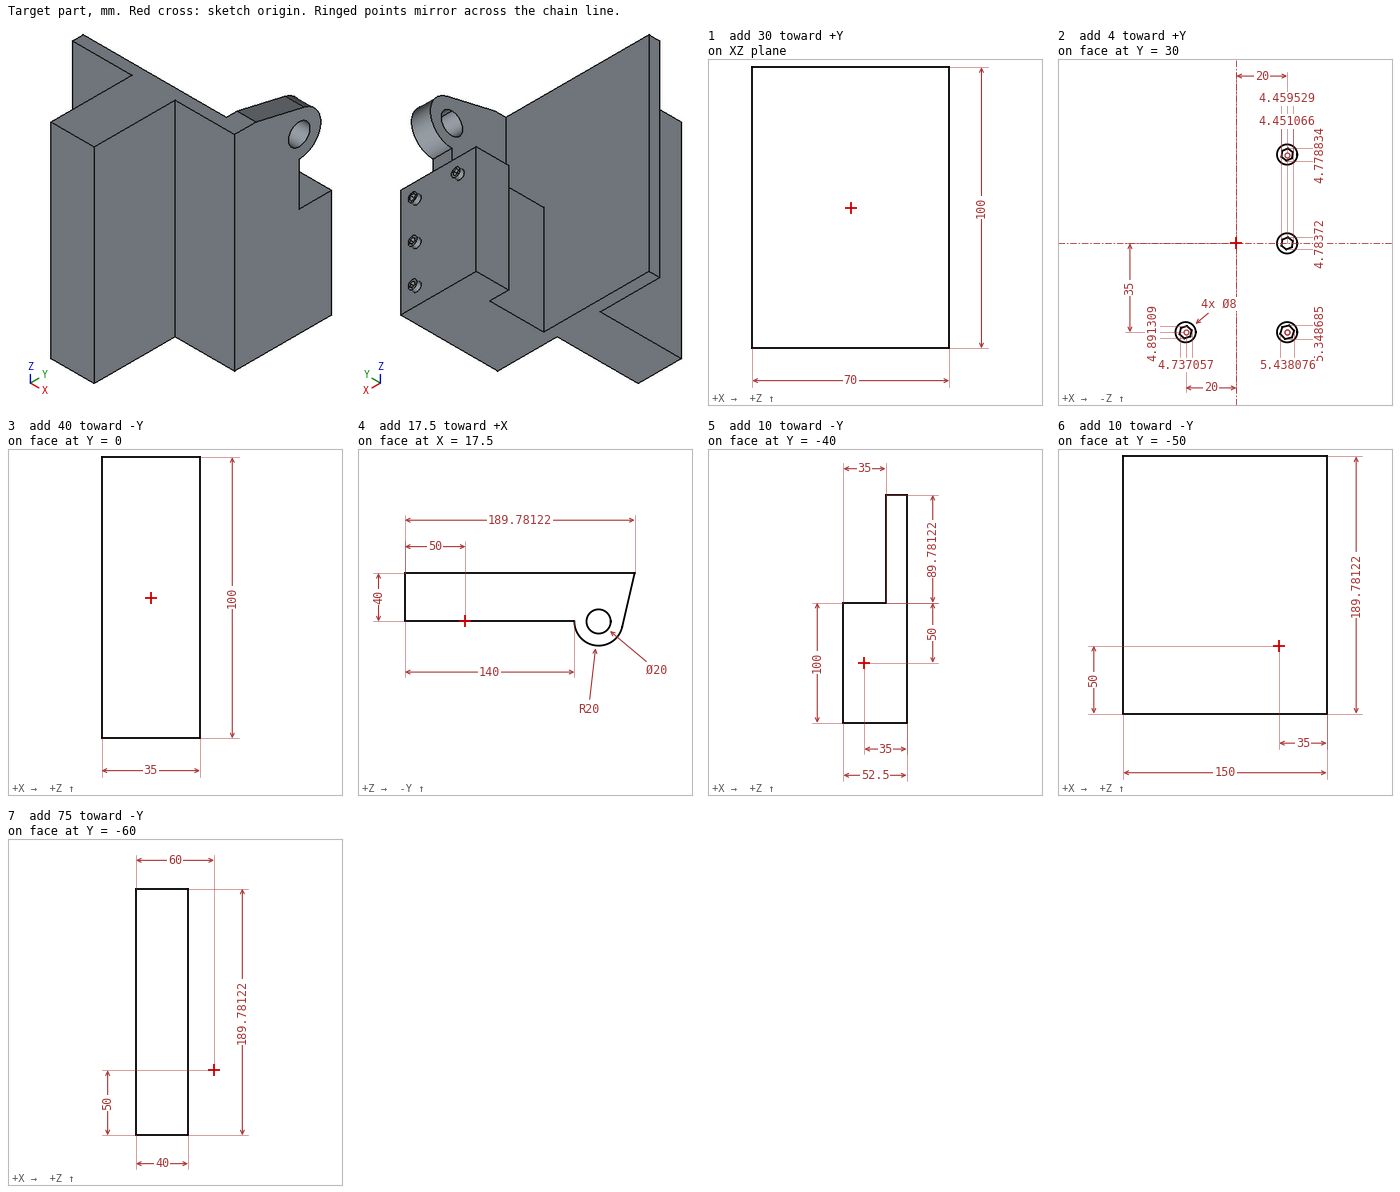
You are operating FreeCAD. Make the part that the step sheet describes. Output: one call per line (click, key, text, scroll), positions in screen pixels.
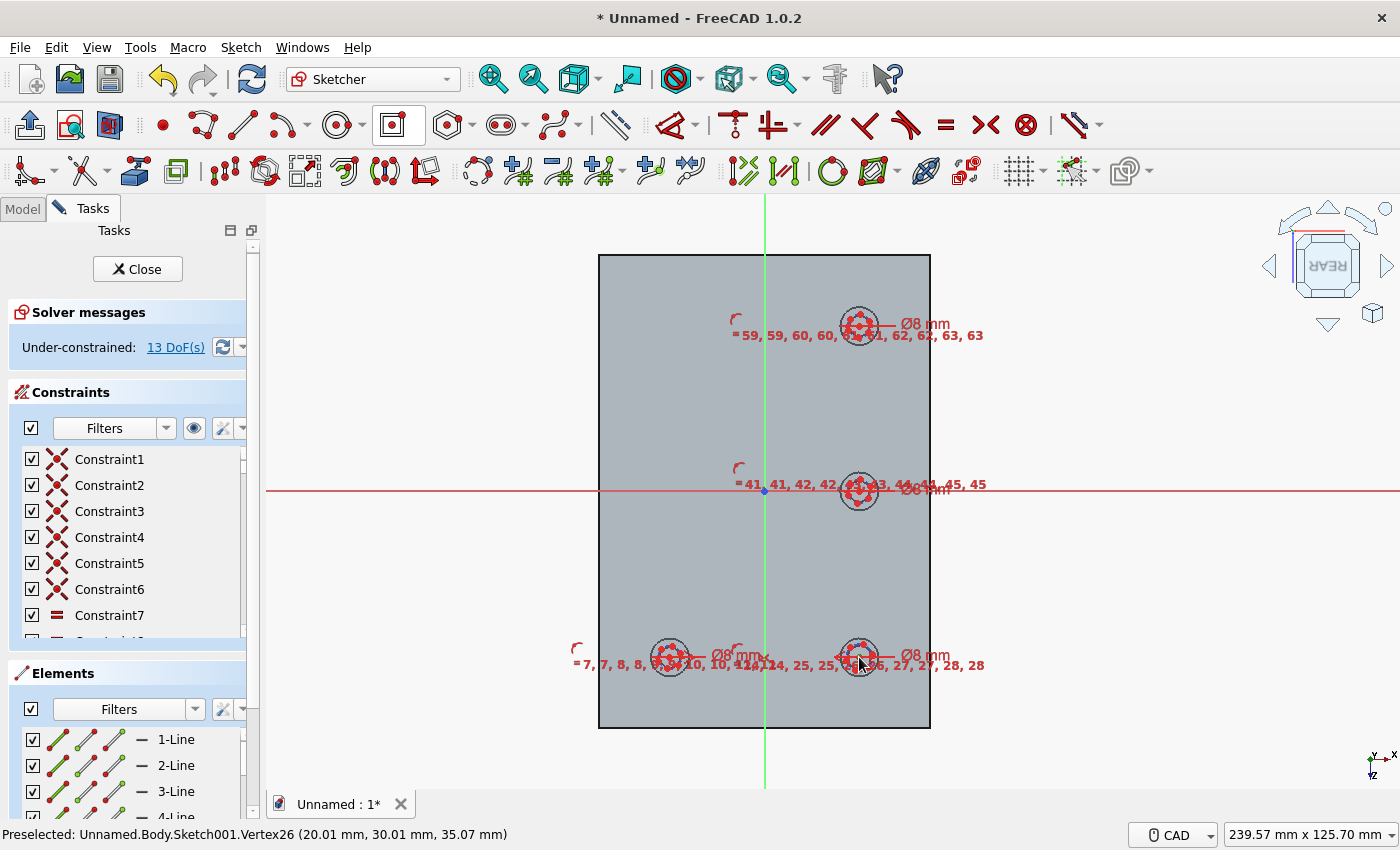
click(859, 326)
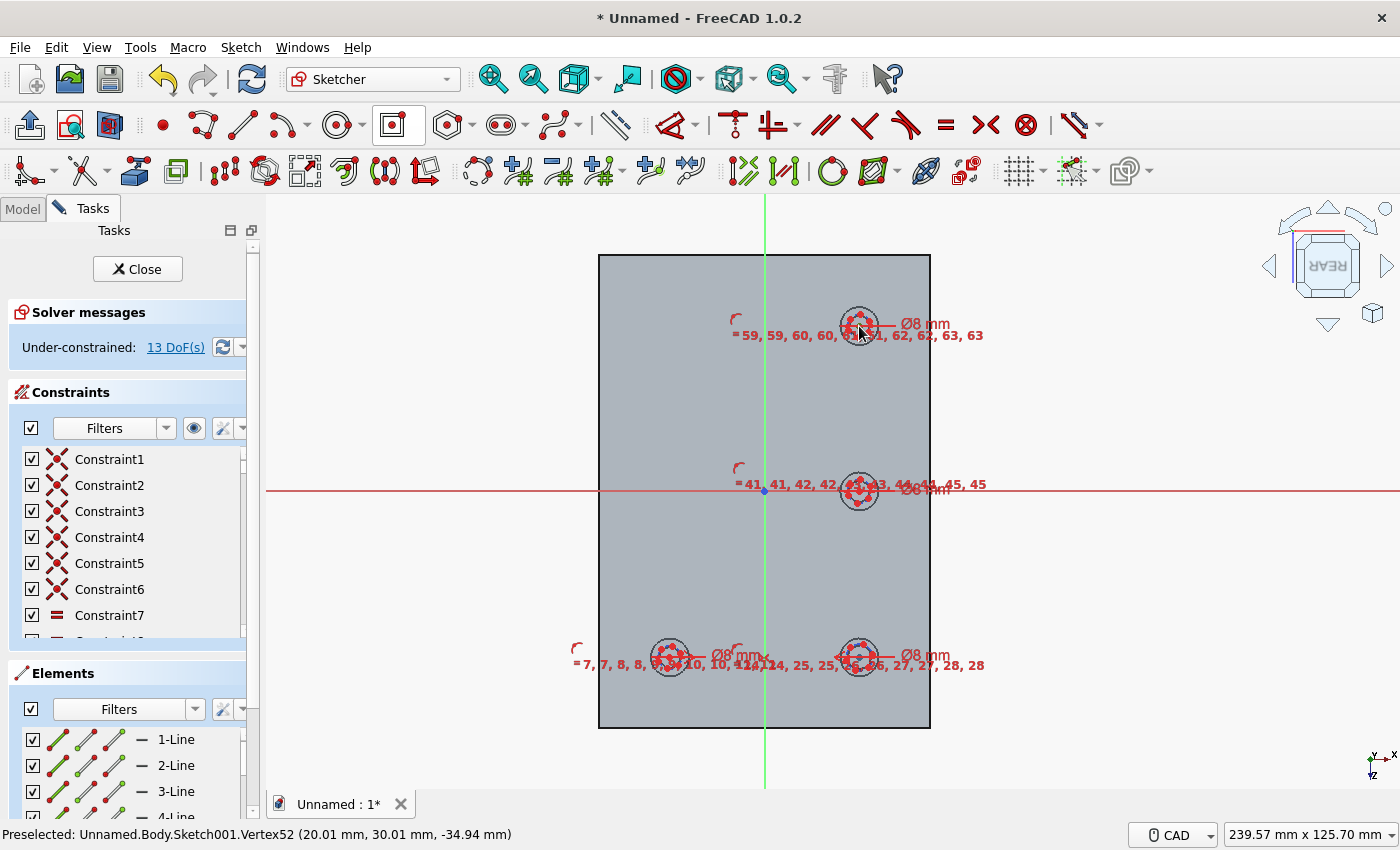
click(361, 491)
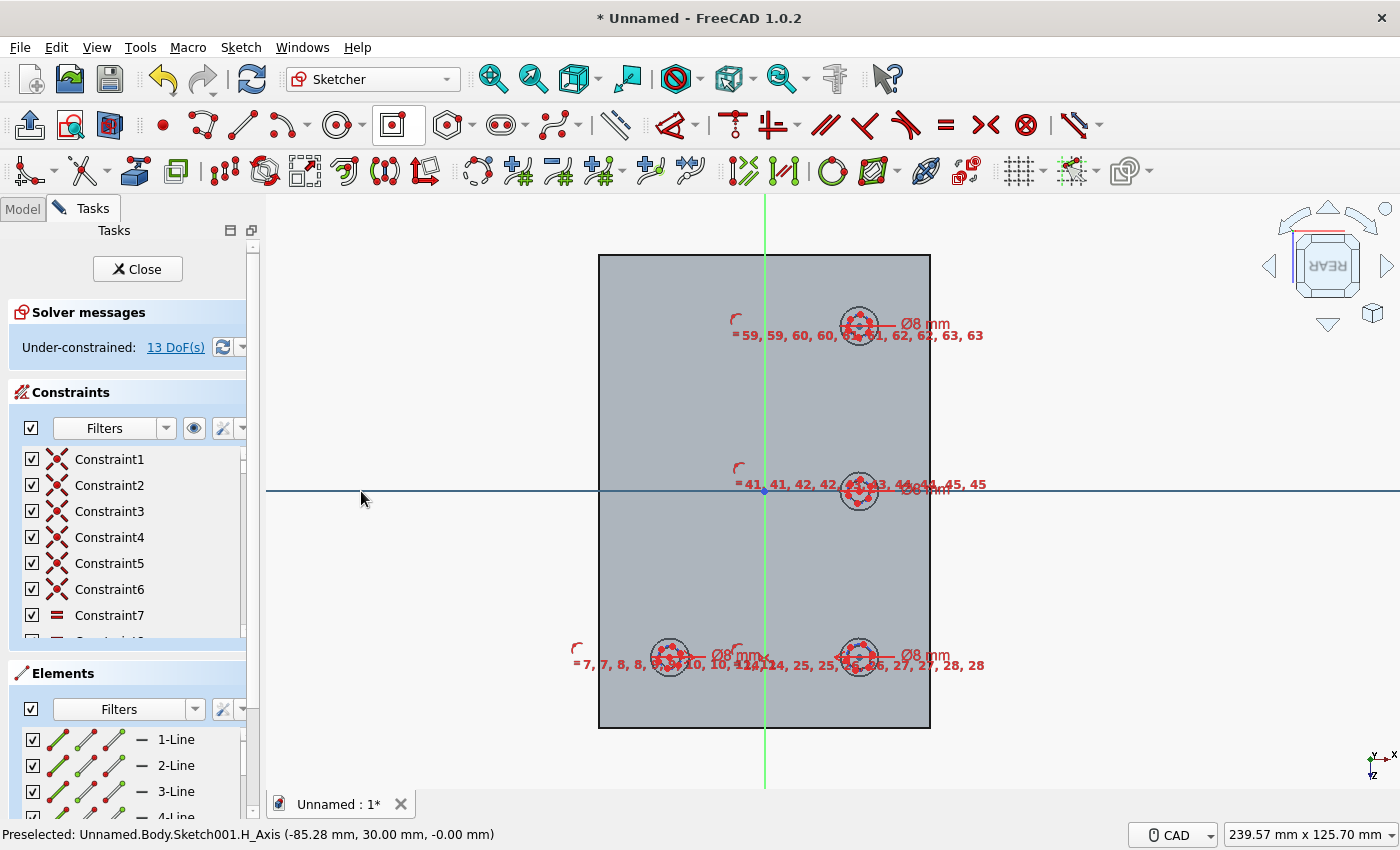
click(986, 126)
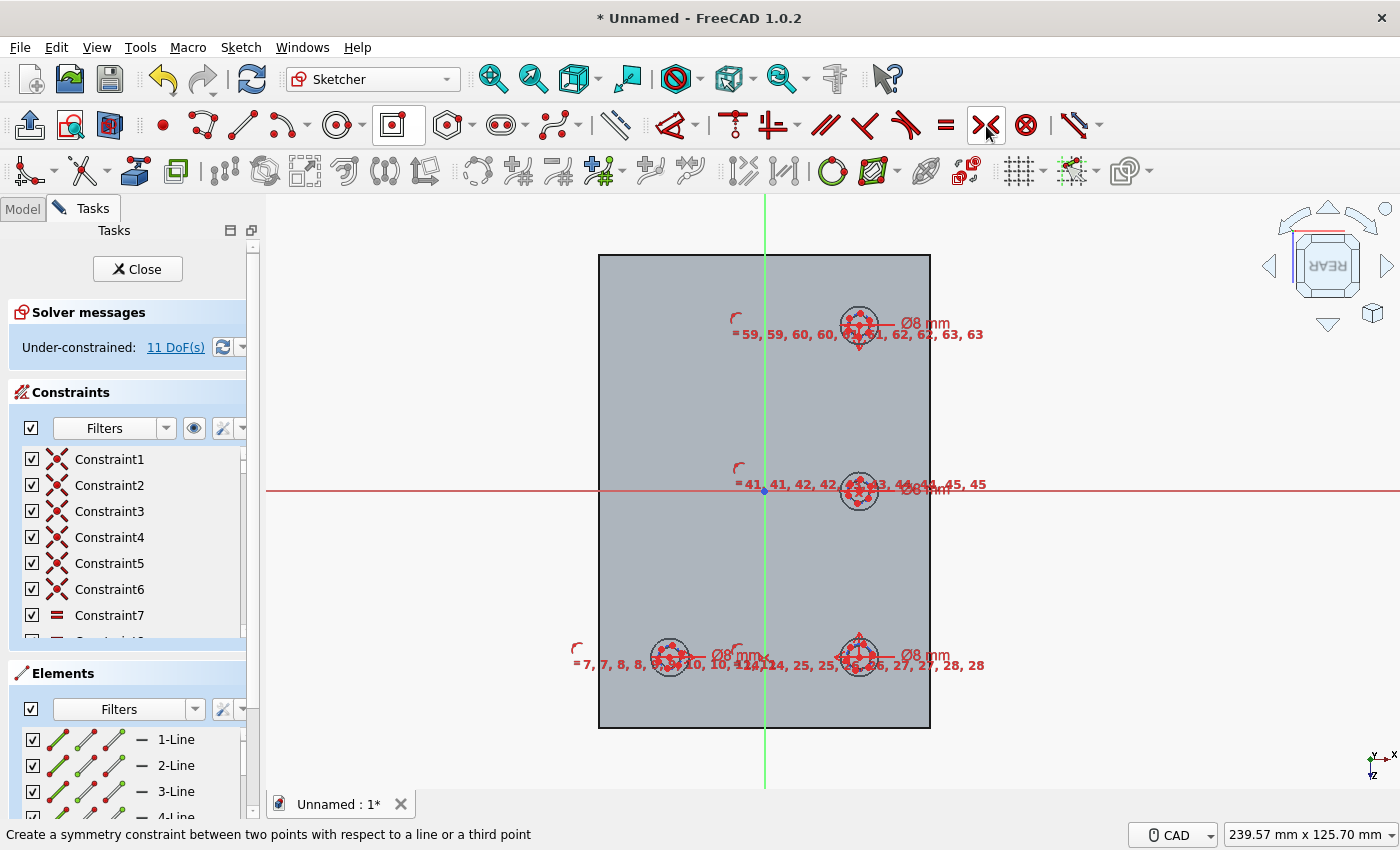
click(670, 126)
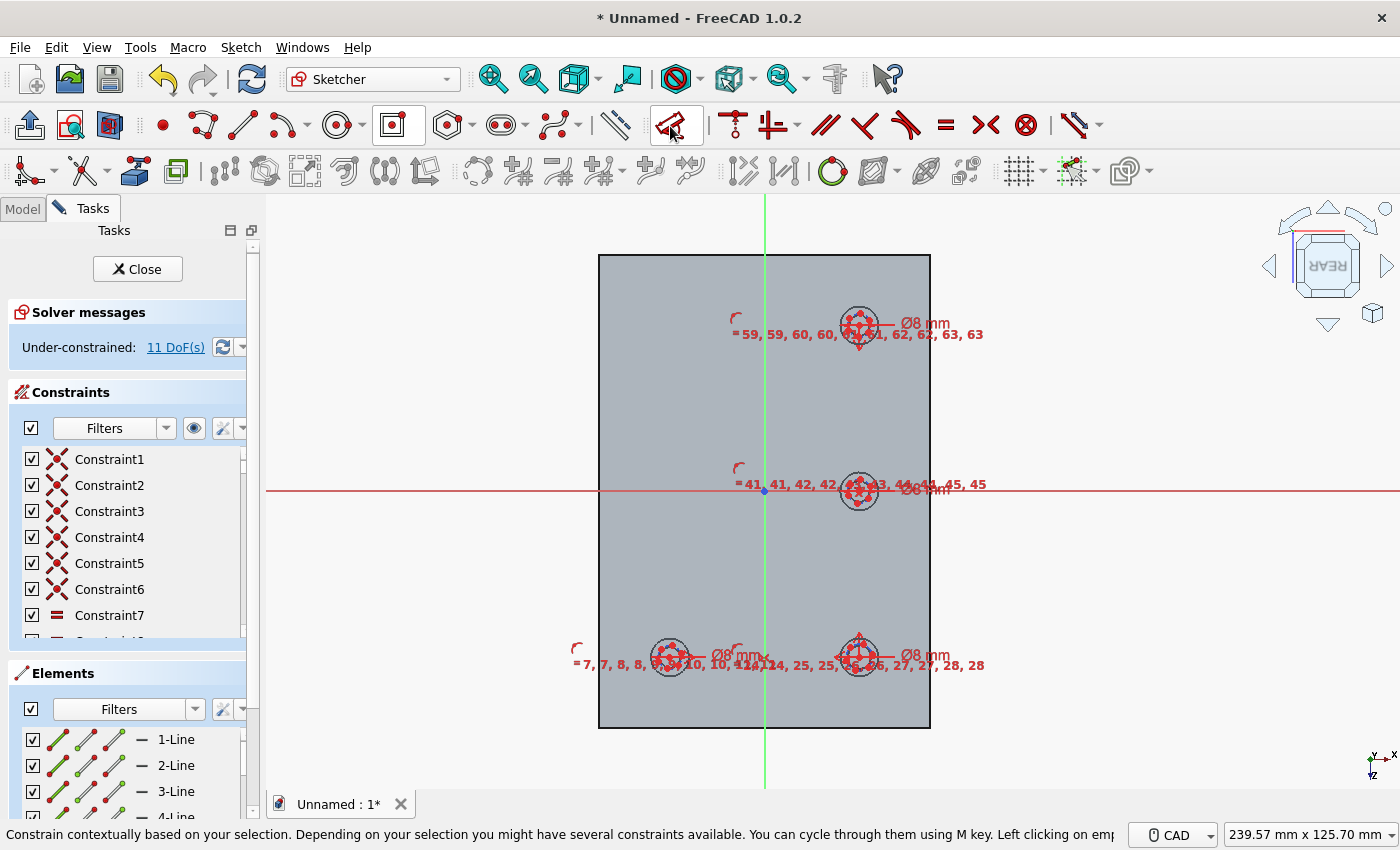
click(670, 657)
click(717, 691)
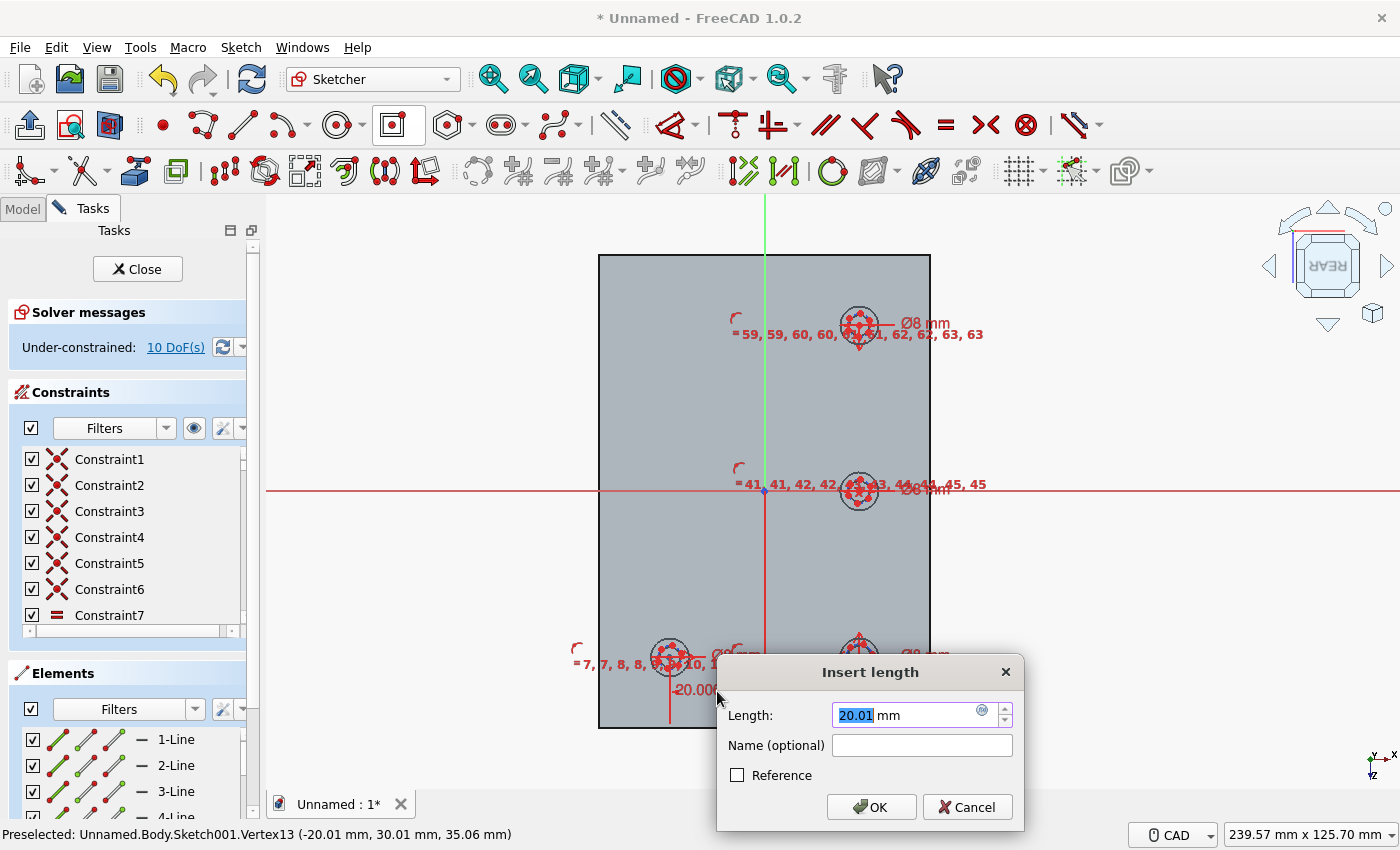
text(20)
key(Return)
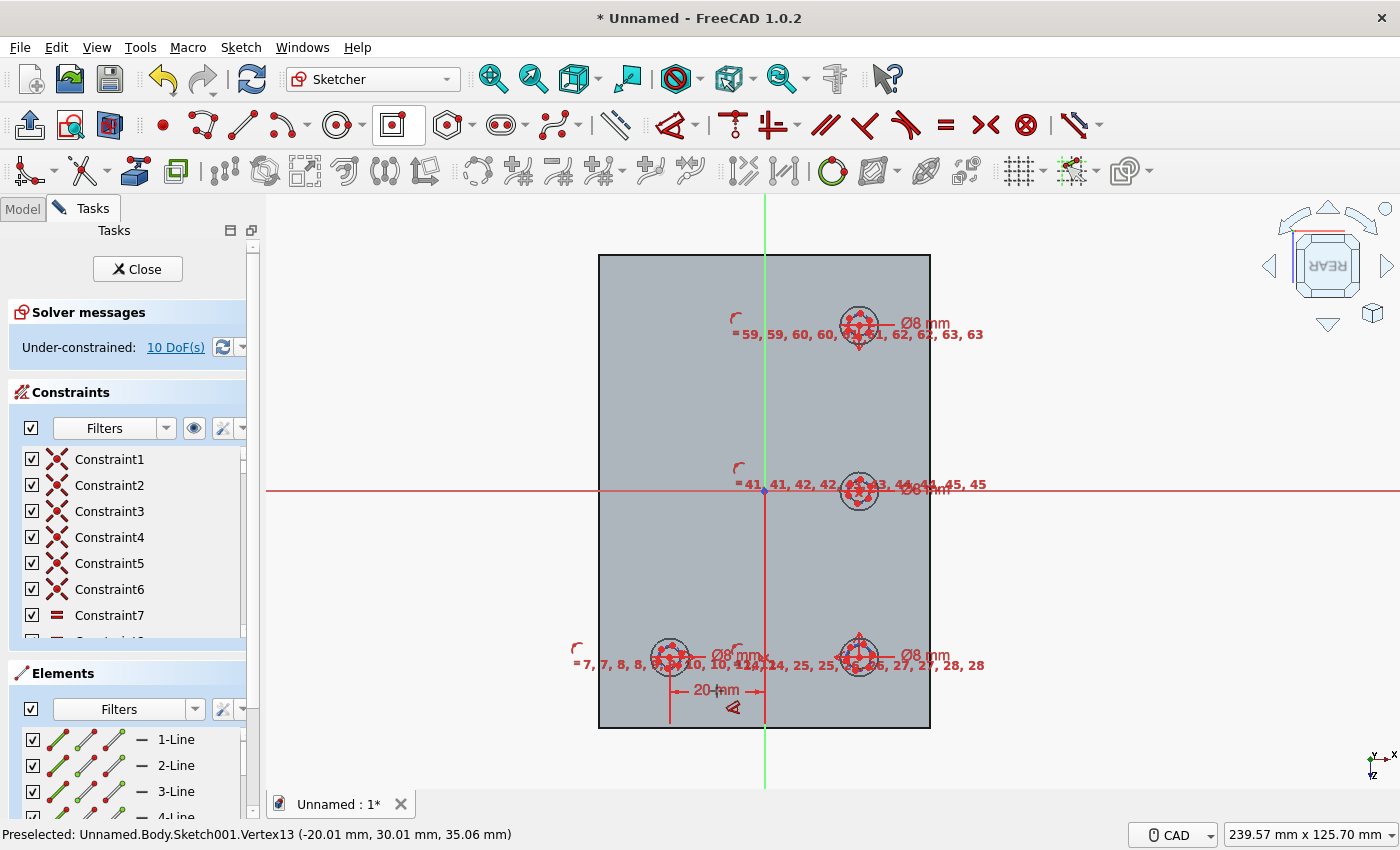
click(670, 657)
click(636, 574)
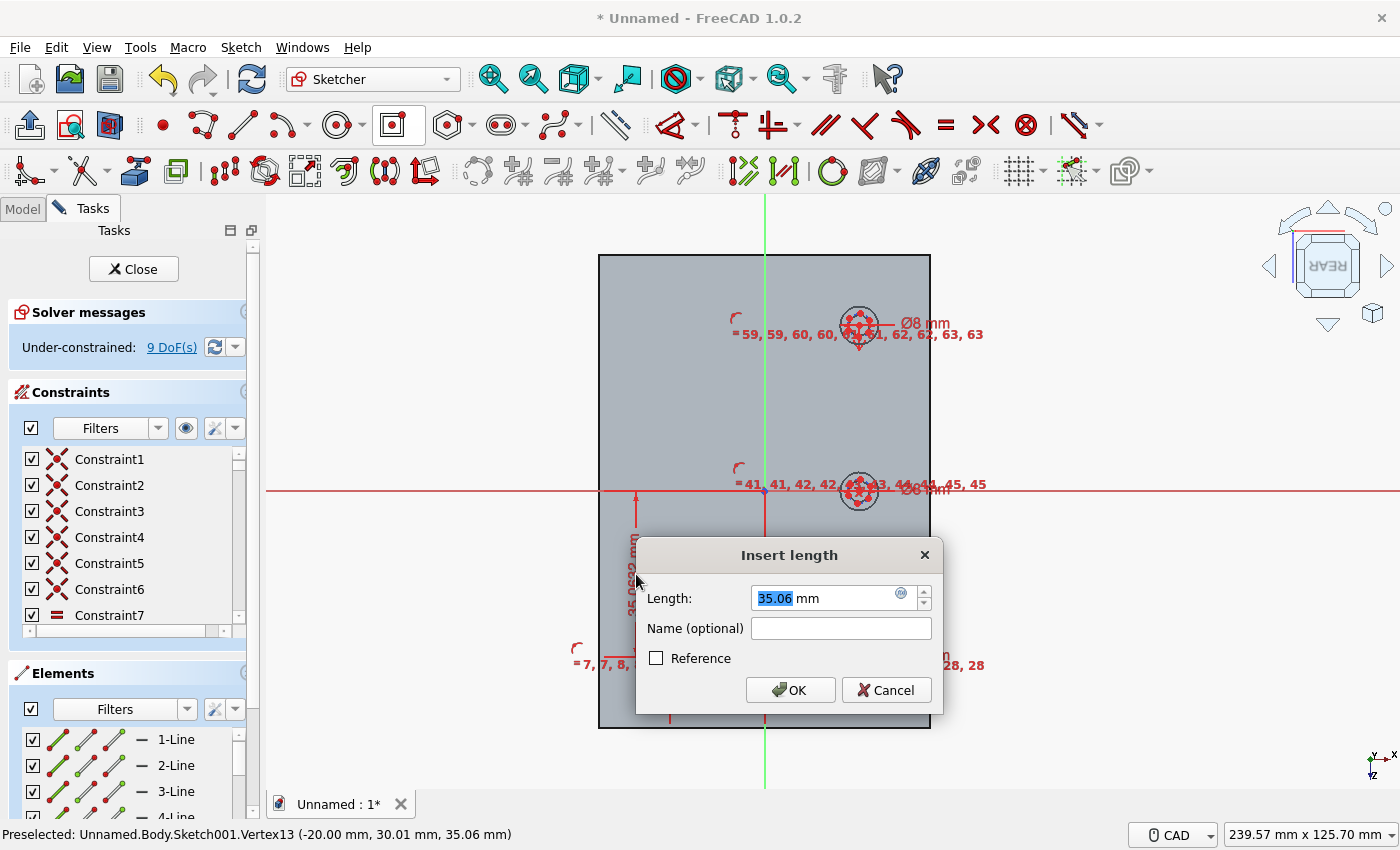
text(35)
key(Return)